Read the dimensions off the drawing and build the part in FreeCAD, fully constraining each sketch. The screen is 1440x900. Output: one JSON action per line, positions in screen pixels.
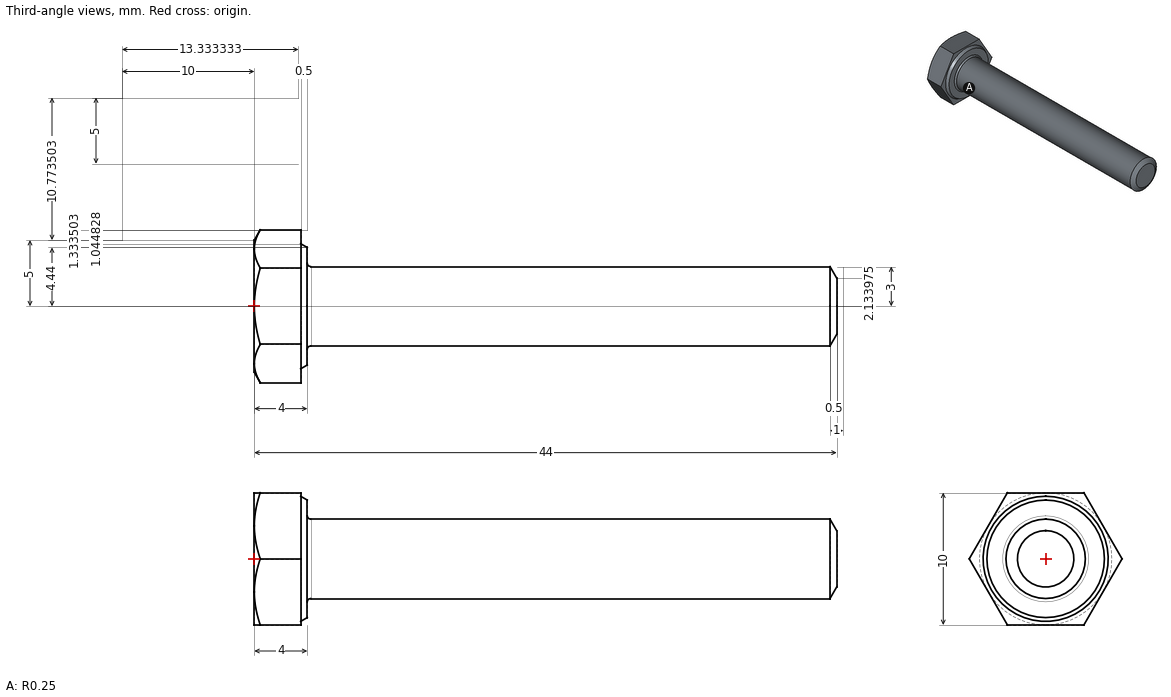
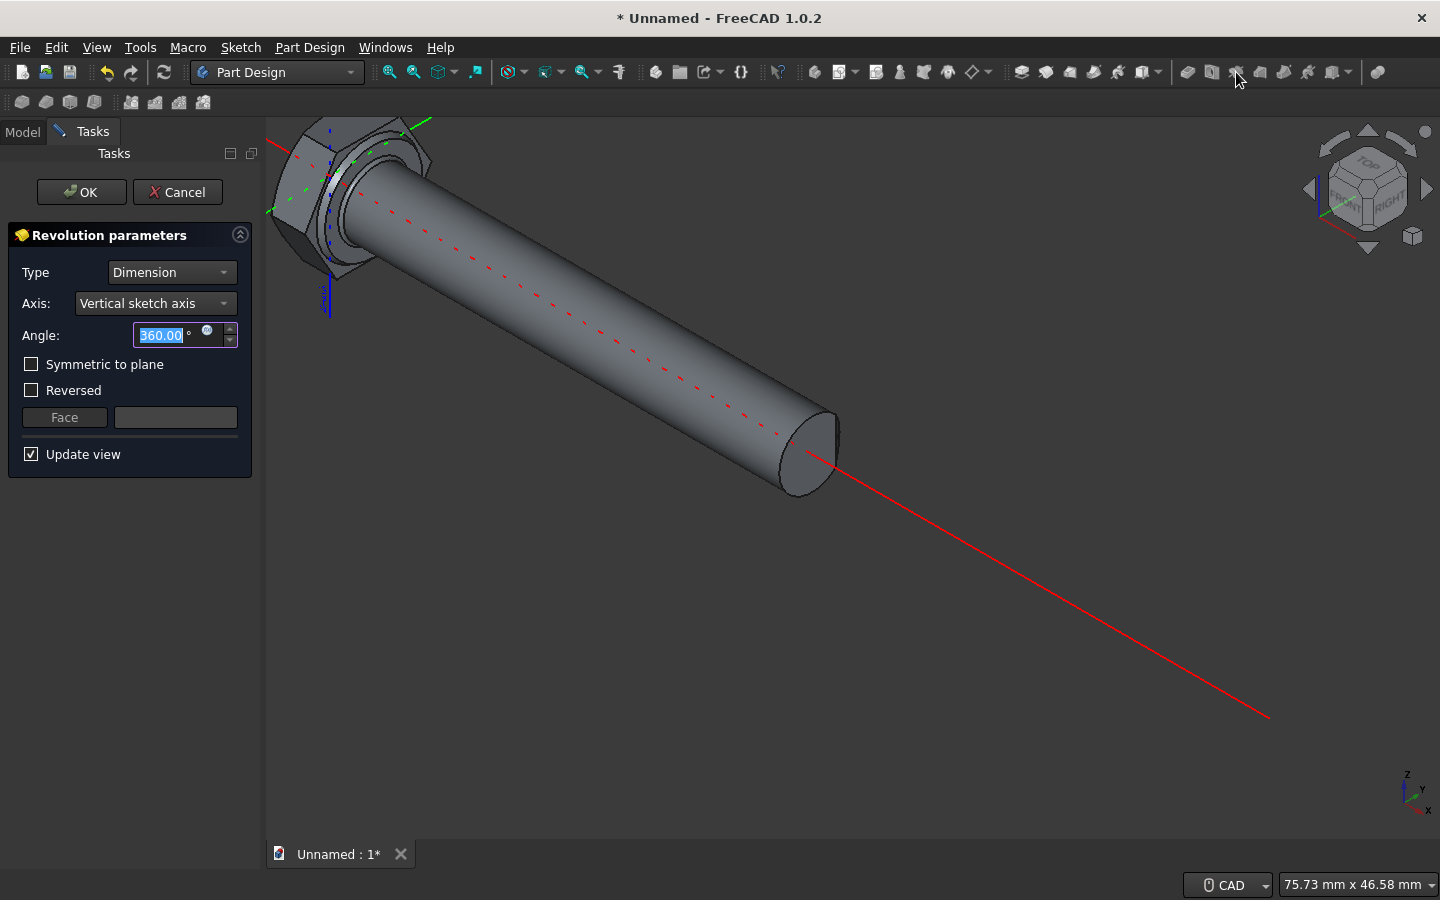
{"action": "left_click", "coordinate": [156, 304]}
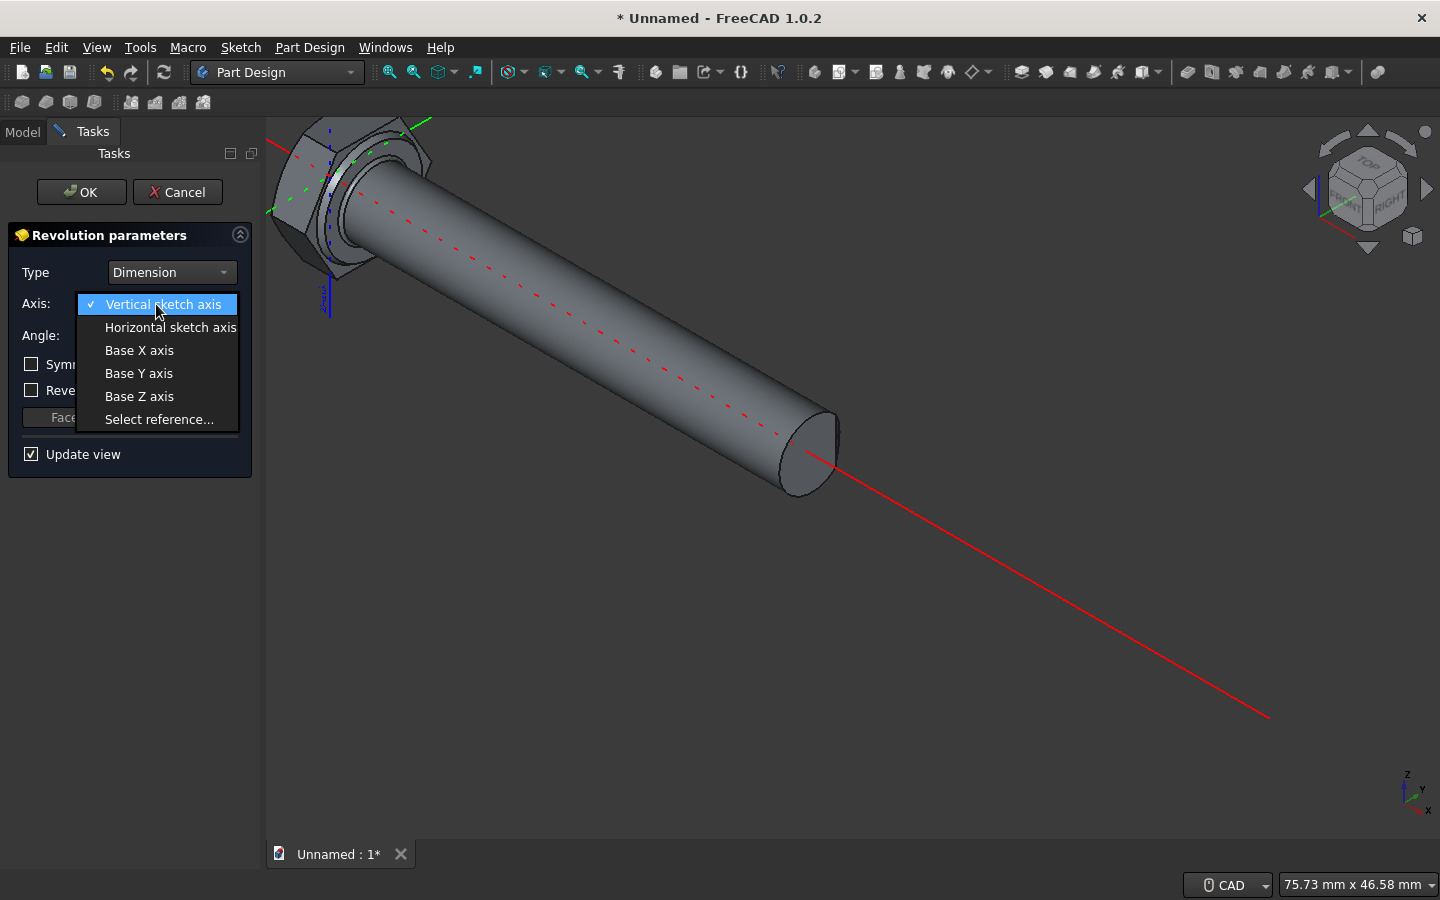
{"action": "left_click", "coordinate": [156, 328]}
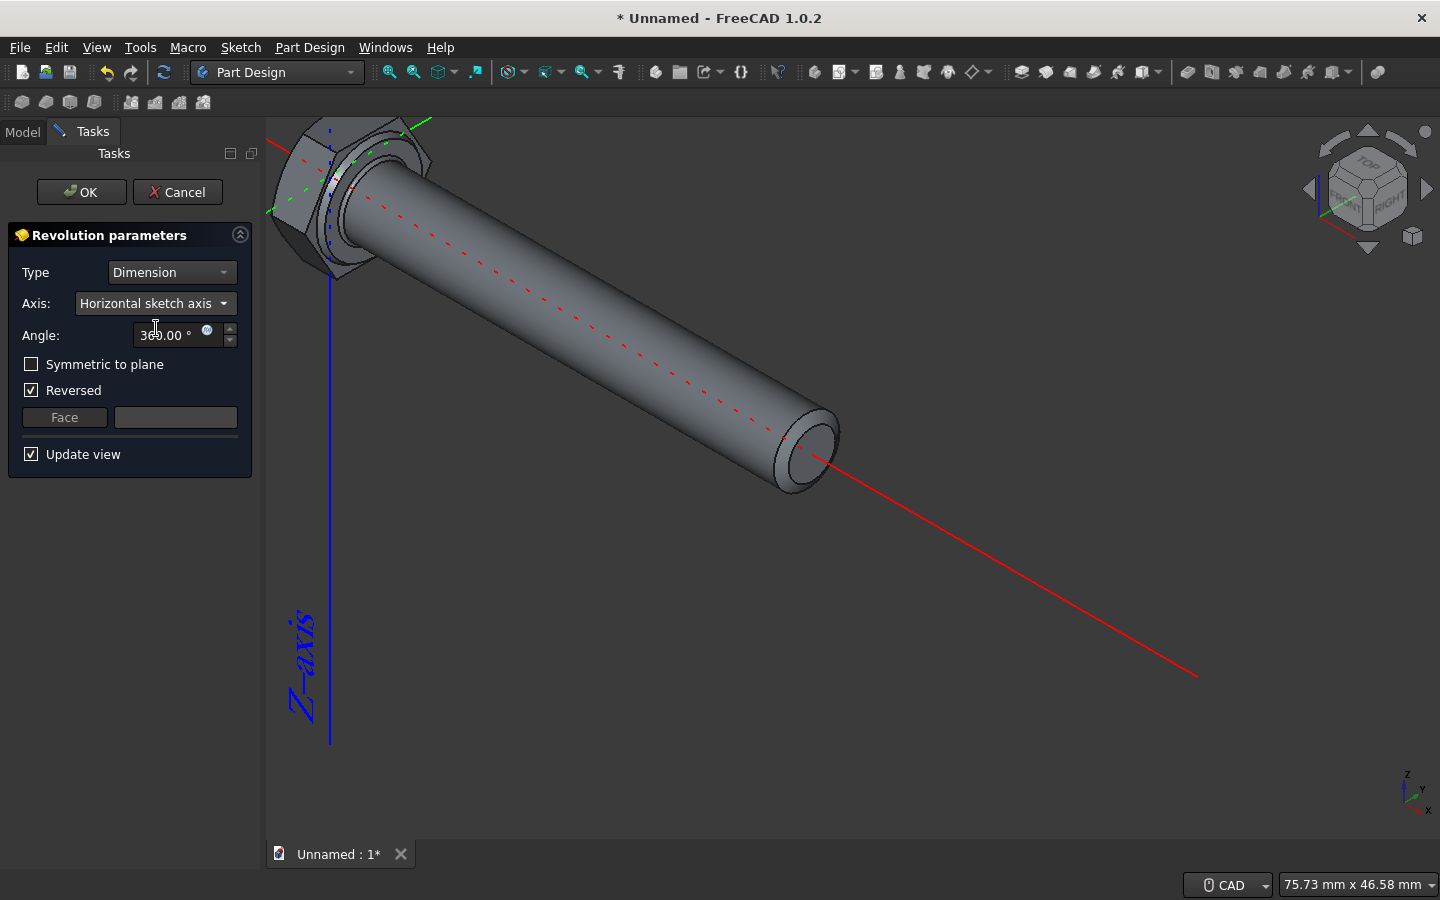
{"action": "left_click", "coordinate": [82, 192]}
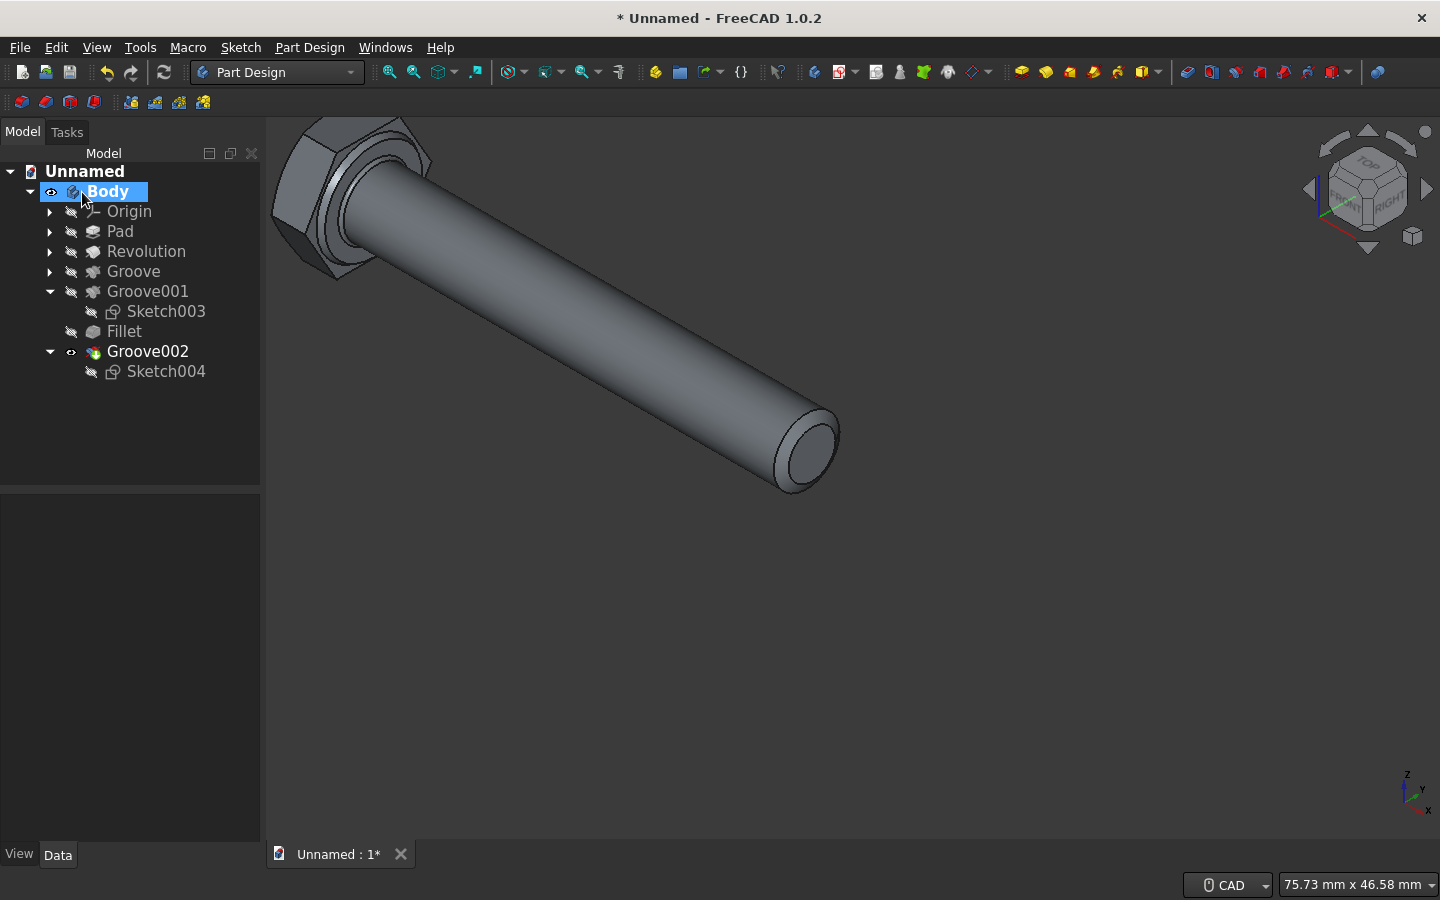
{"action": "left_click", "coordinate": [390, 72]}